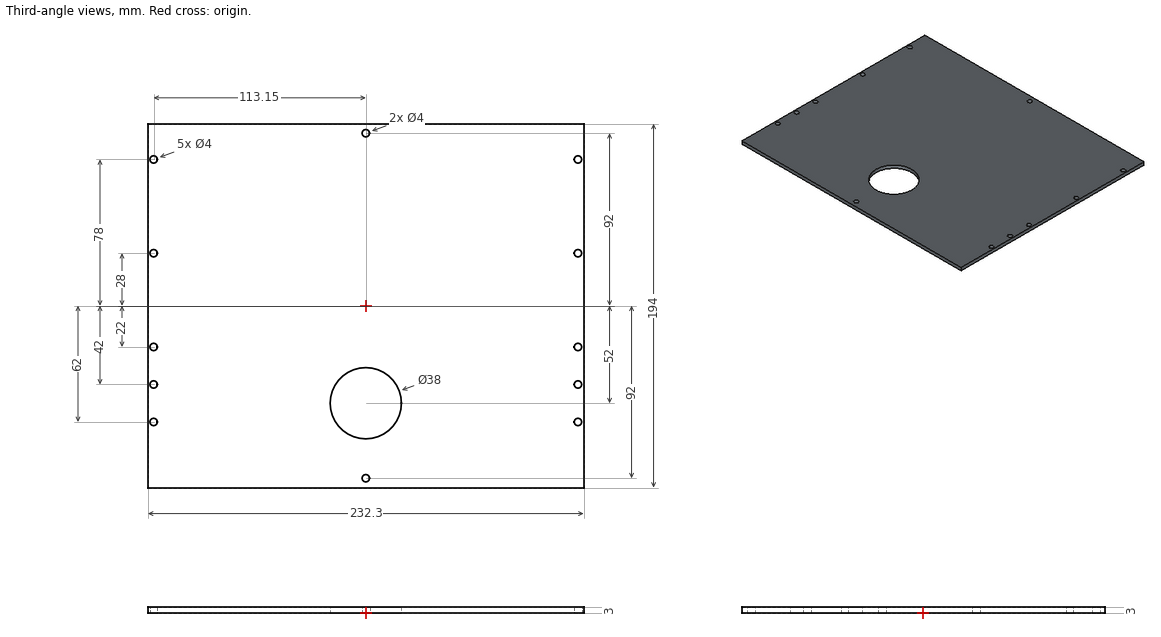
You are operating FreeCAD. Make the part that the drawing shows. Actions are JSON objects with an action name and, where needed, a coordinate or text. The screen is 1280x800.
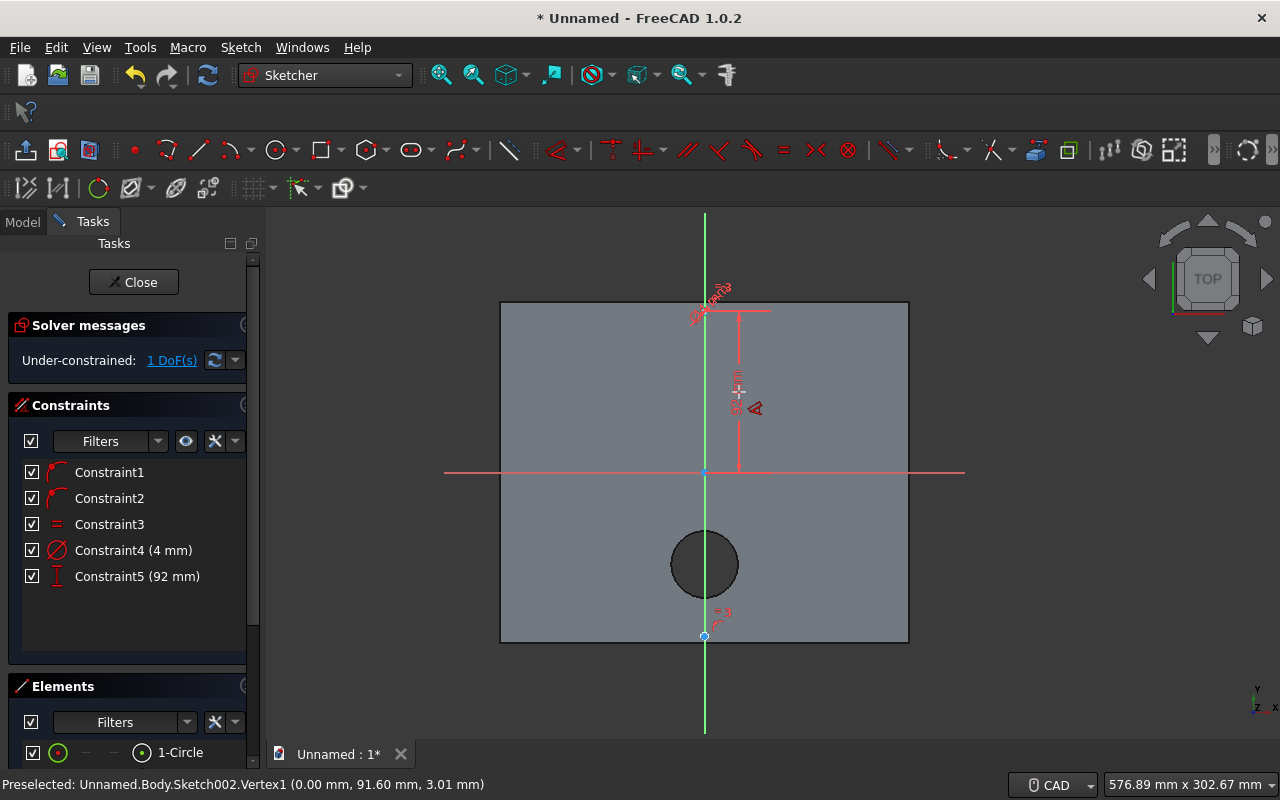
{"action": "left_click", "coordinate": [705, 636]}
{"action": "left_click", "coordinate": [739, 555]}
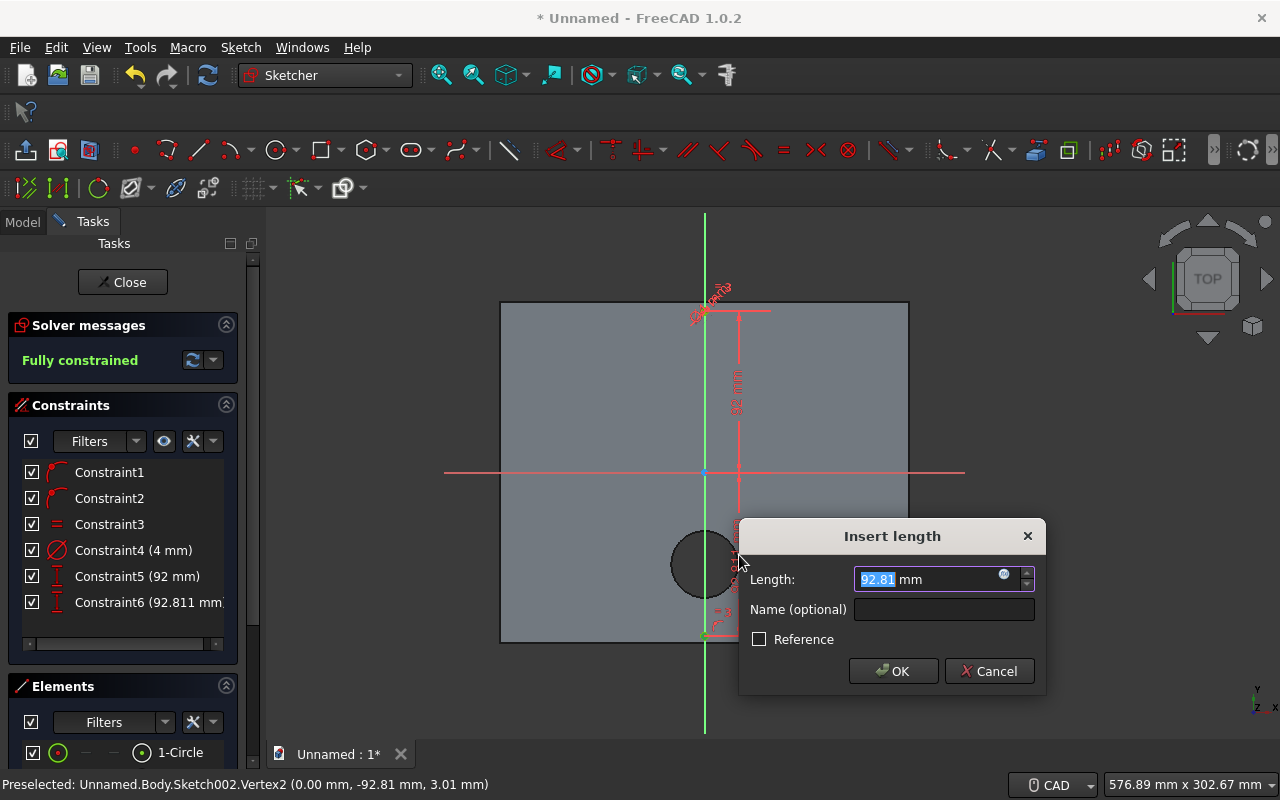
{"action": "type", "text": "92"}
{"action": "key", "text": "Return"}
{"action": "key", "text": "Escape"}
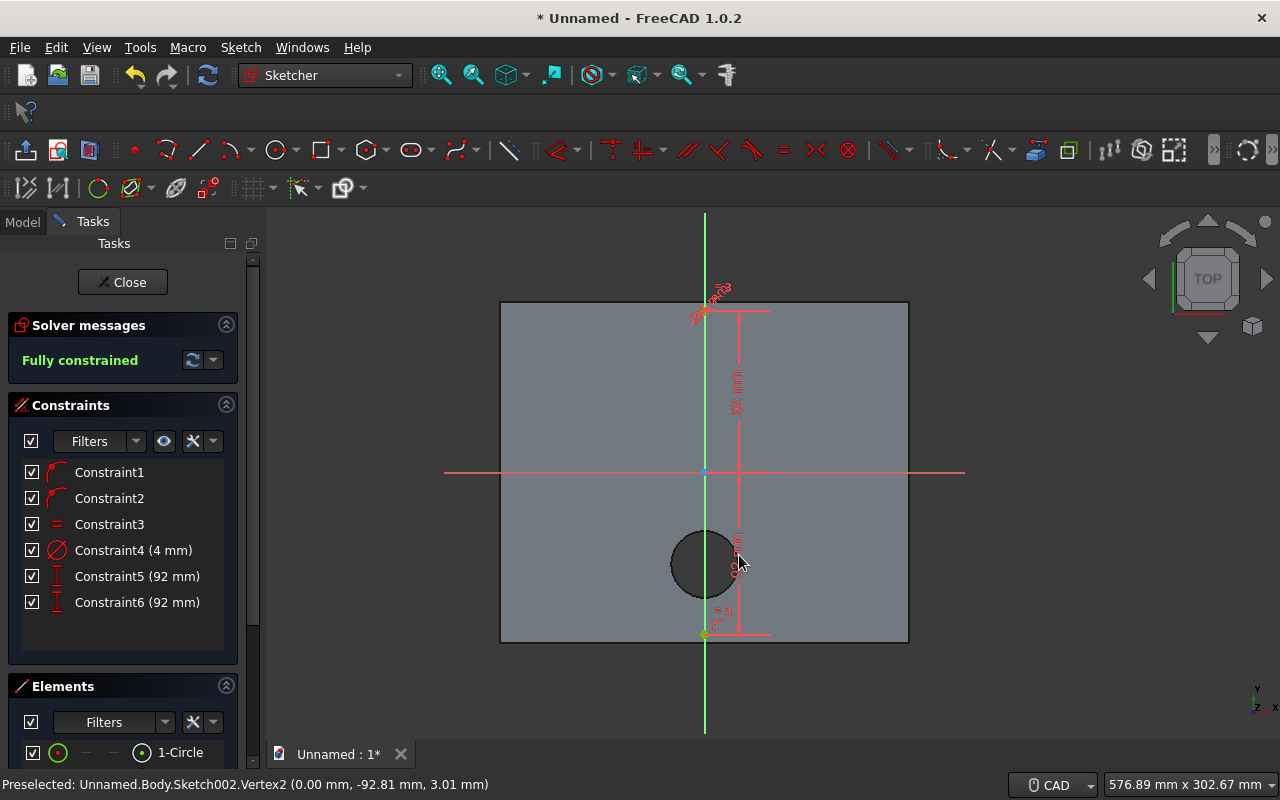
{"action": "left_click", "coordinate": [123, 282]}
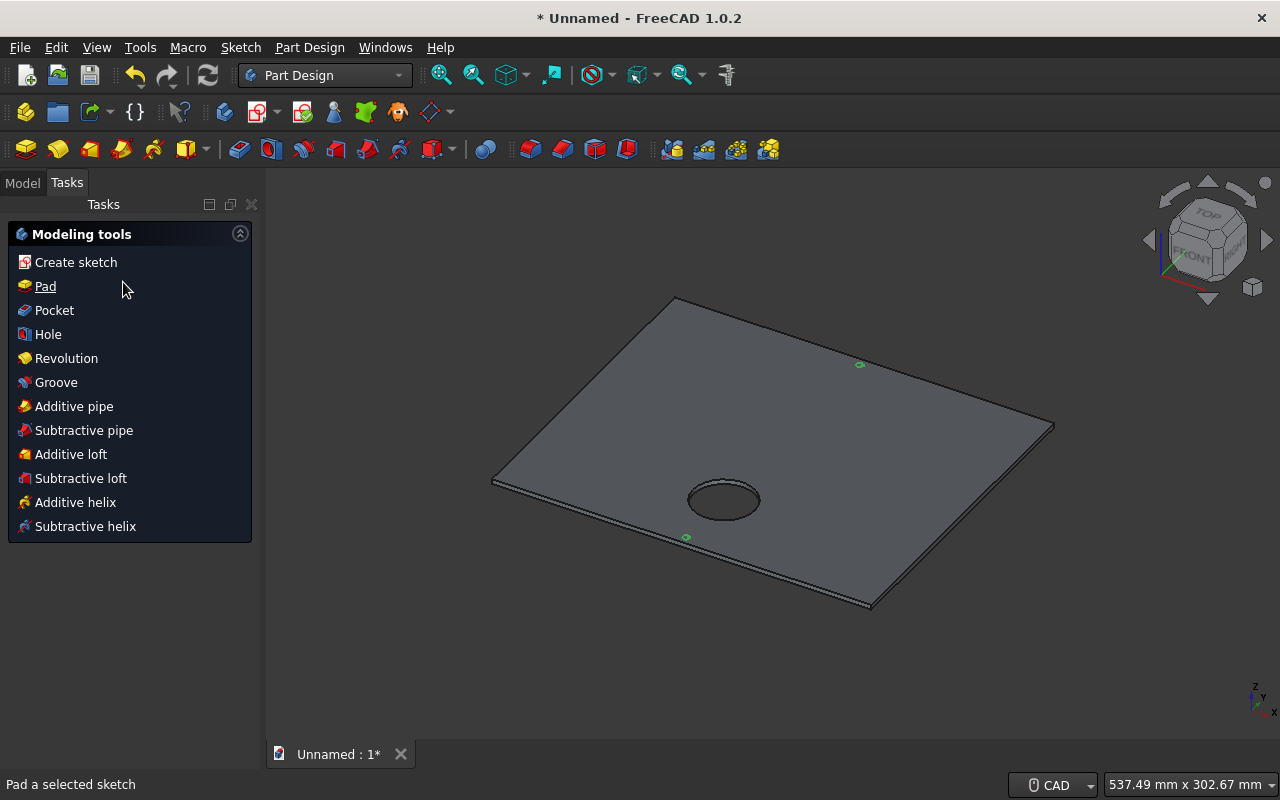
{"action": "left_click", "coordinate": [240, 150]}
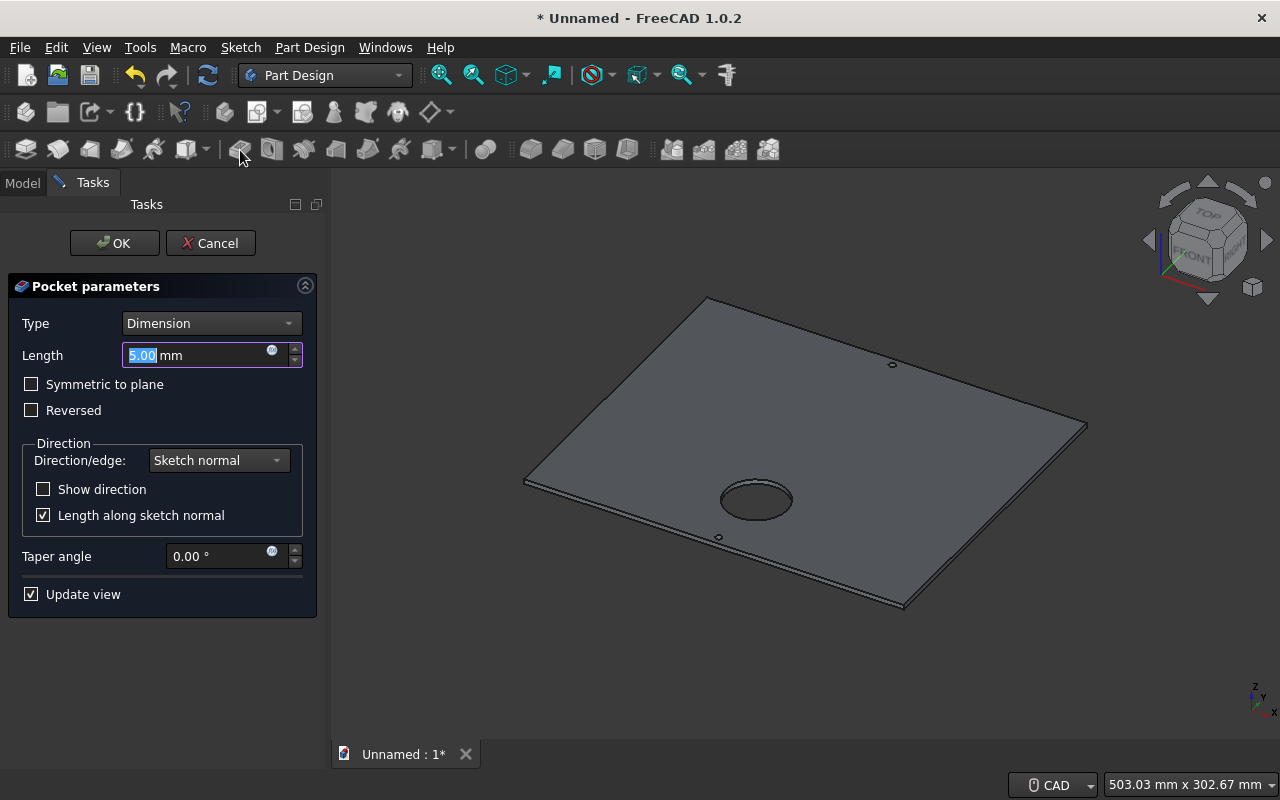
{"action": "type", "text": "4"}
{"action": "key", "text": "Tab"}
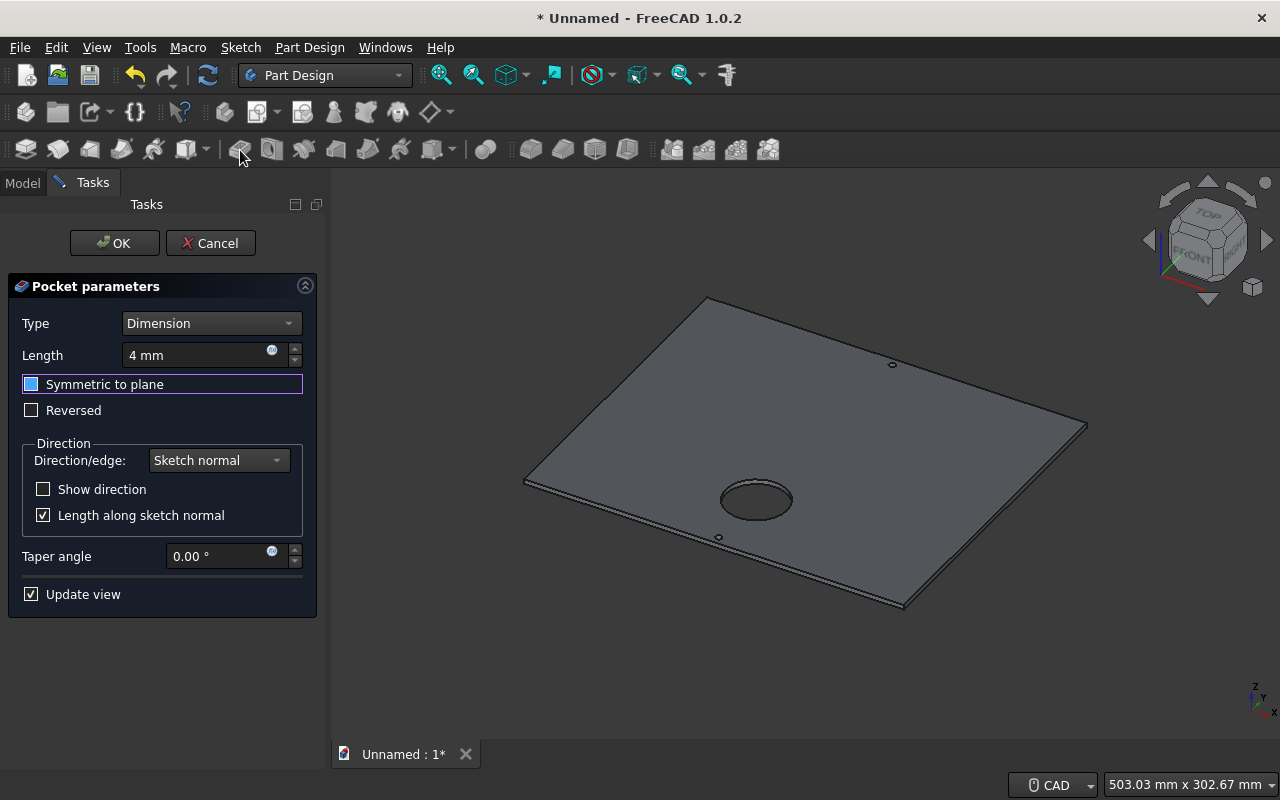
{"action": "left_click", "coordinate": [115, 243]}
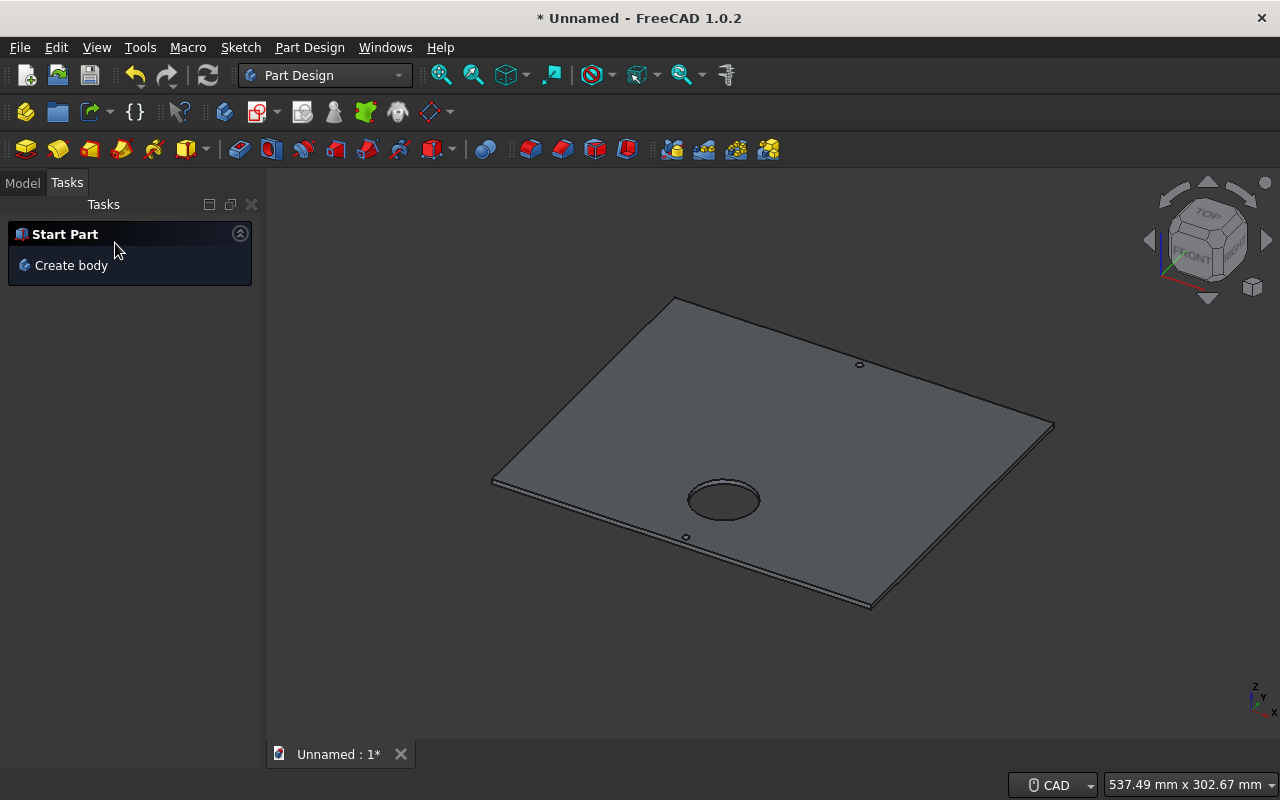
{"action": "left_click", "coordinate": [853, 442]}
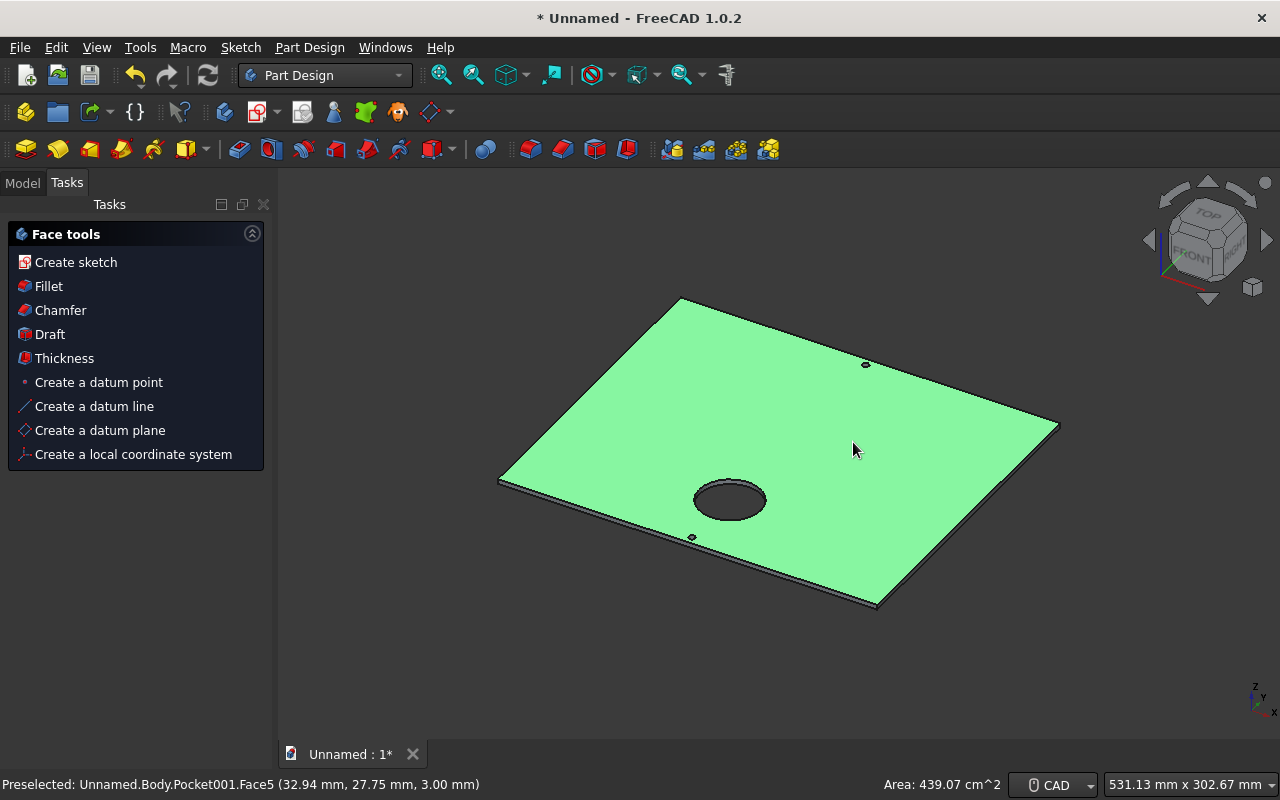
{"action": "left_click", "coordinate": [258, 112]}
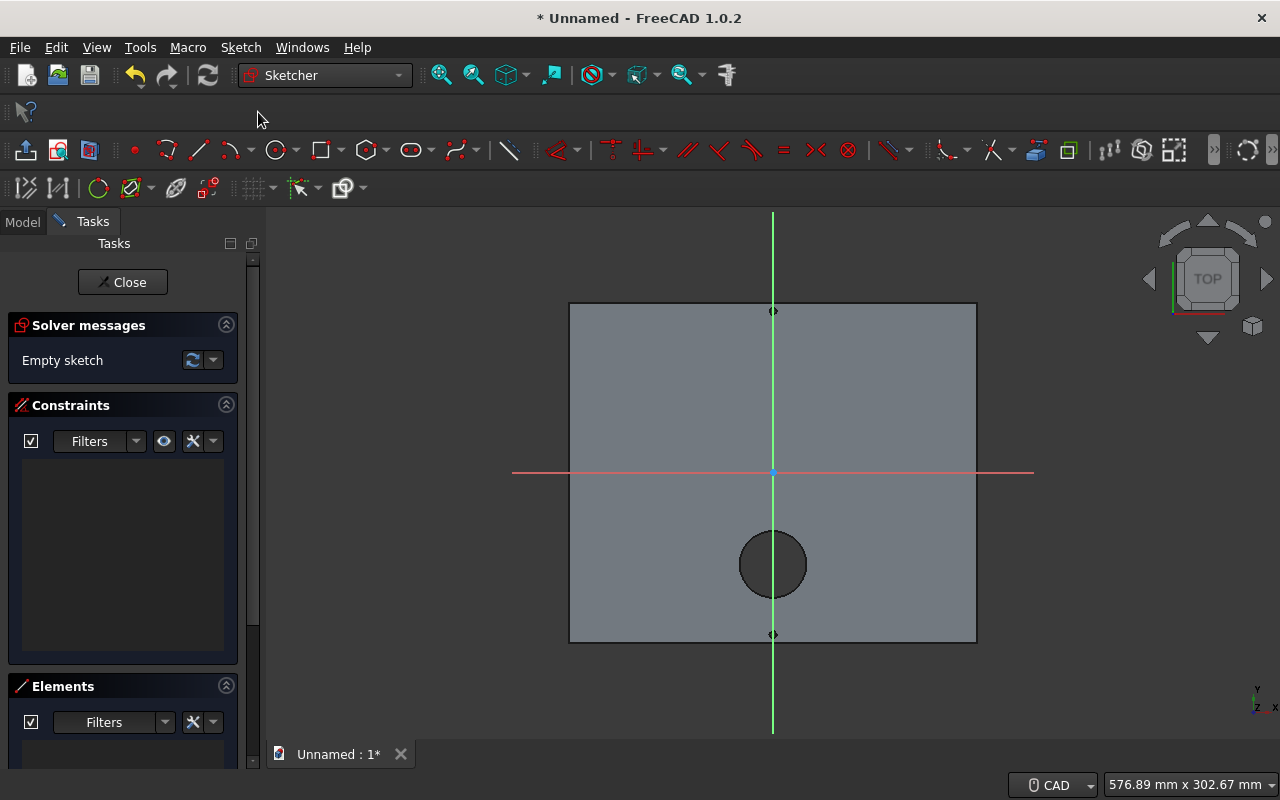
{"action": "key", "text": "g c"}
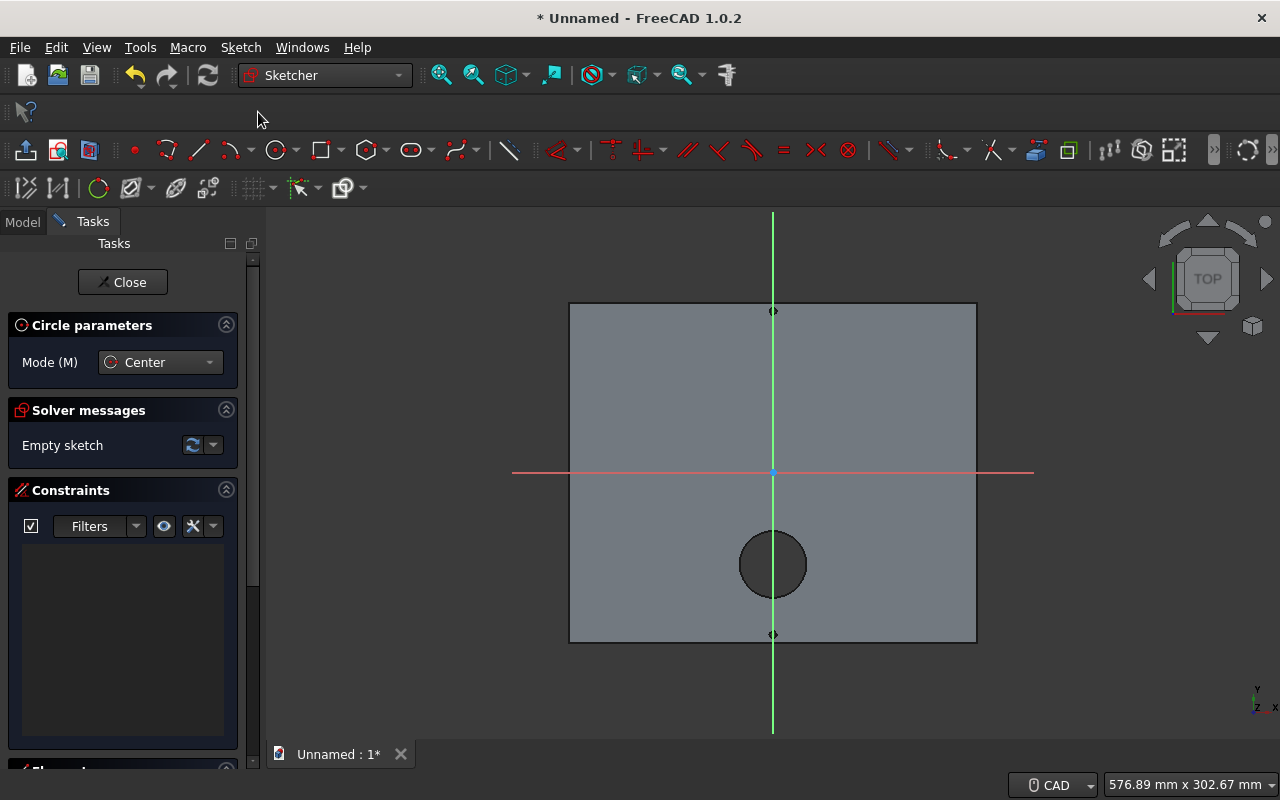
{"action": "scroll", "coordinate": [574, 336], "scroll_direction": "up", "scroll_amount": 10}